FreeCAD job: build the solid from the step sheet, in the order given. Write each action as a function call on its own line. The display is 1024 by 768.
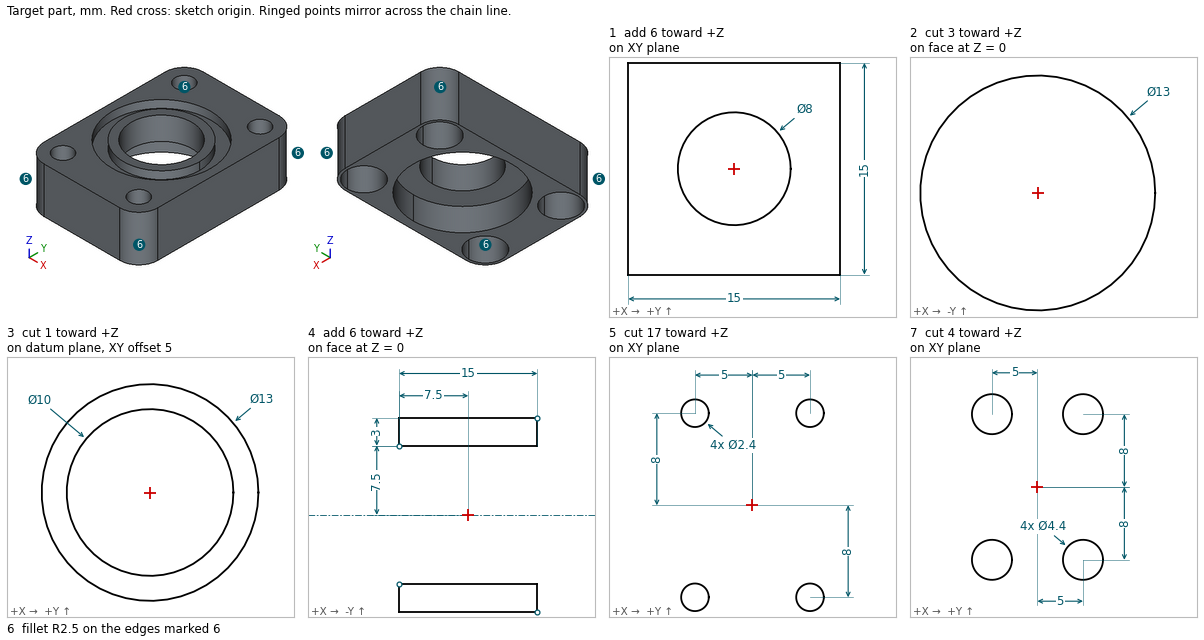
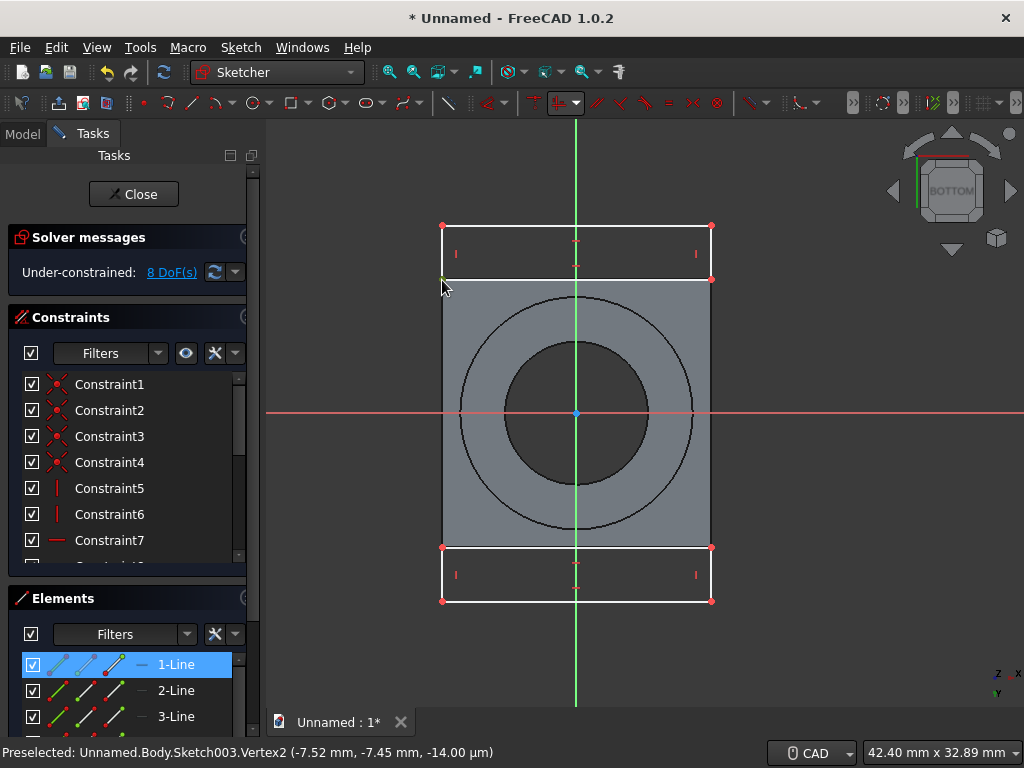
click(442, 548)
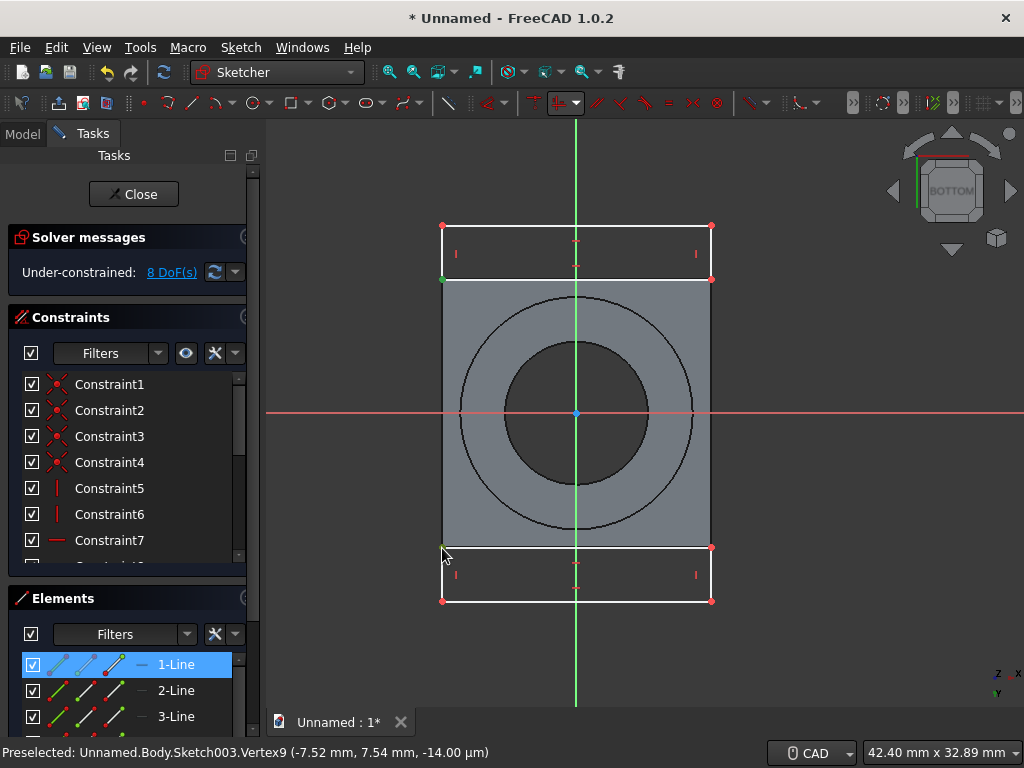
click(334, 413)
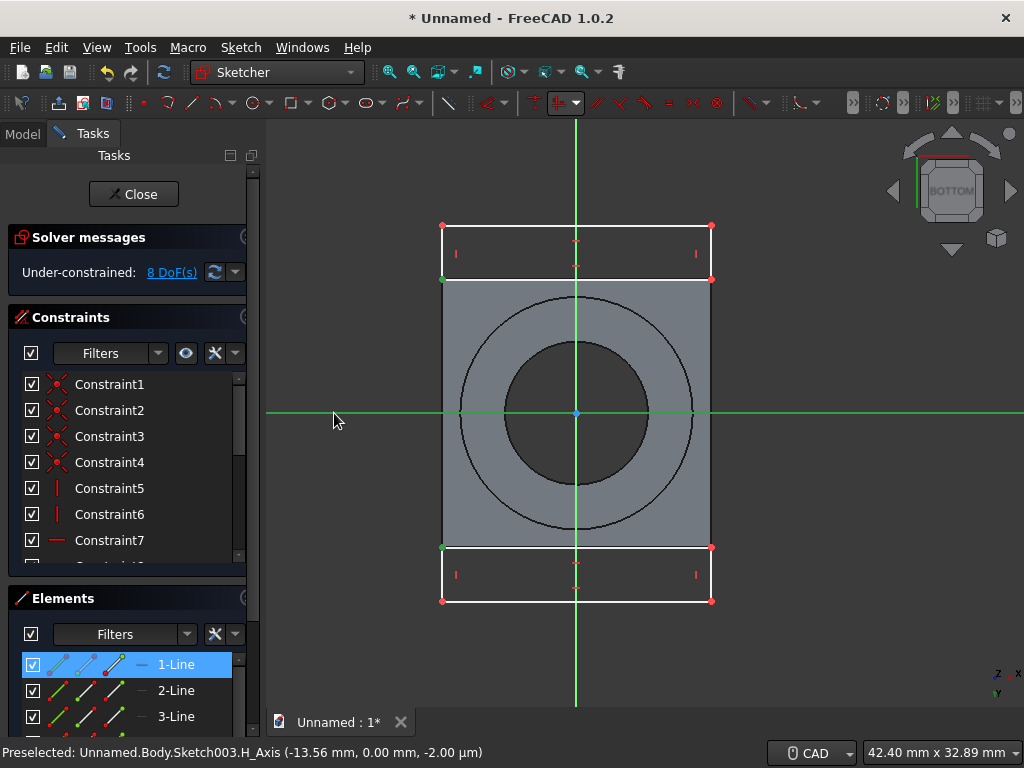
click(694, 104)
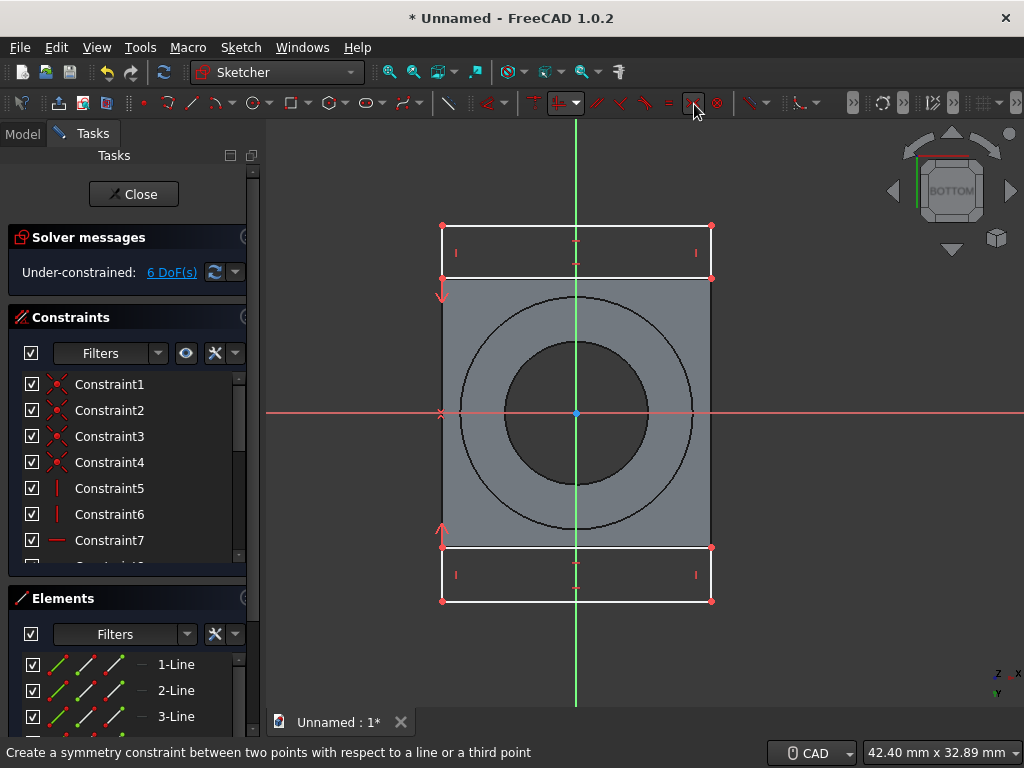
click(711, 226)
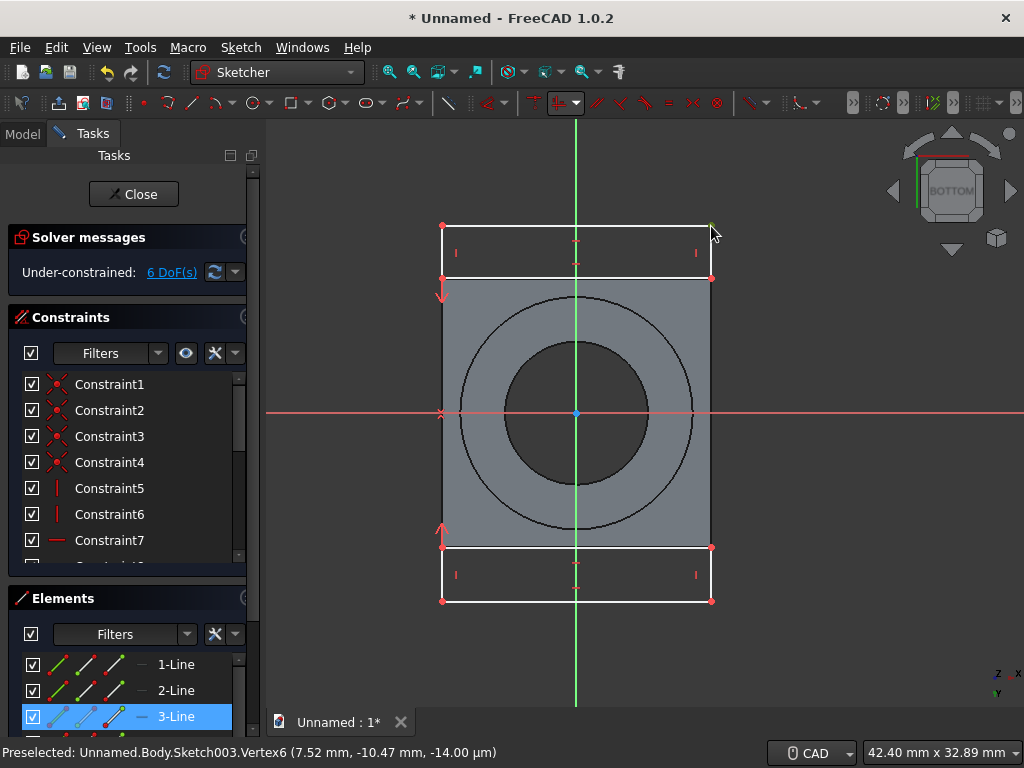
click(711, 602)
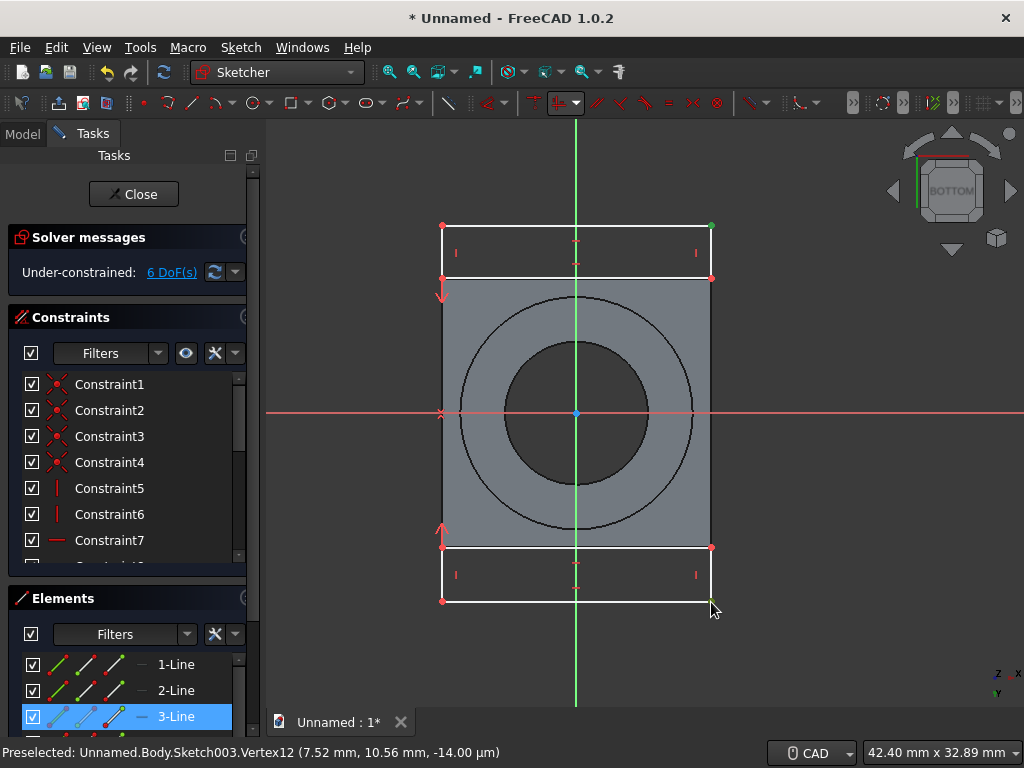
click(334, 413)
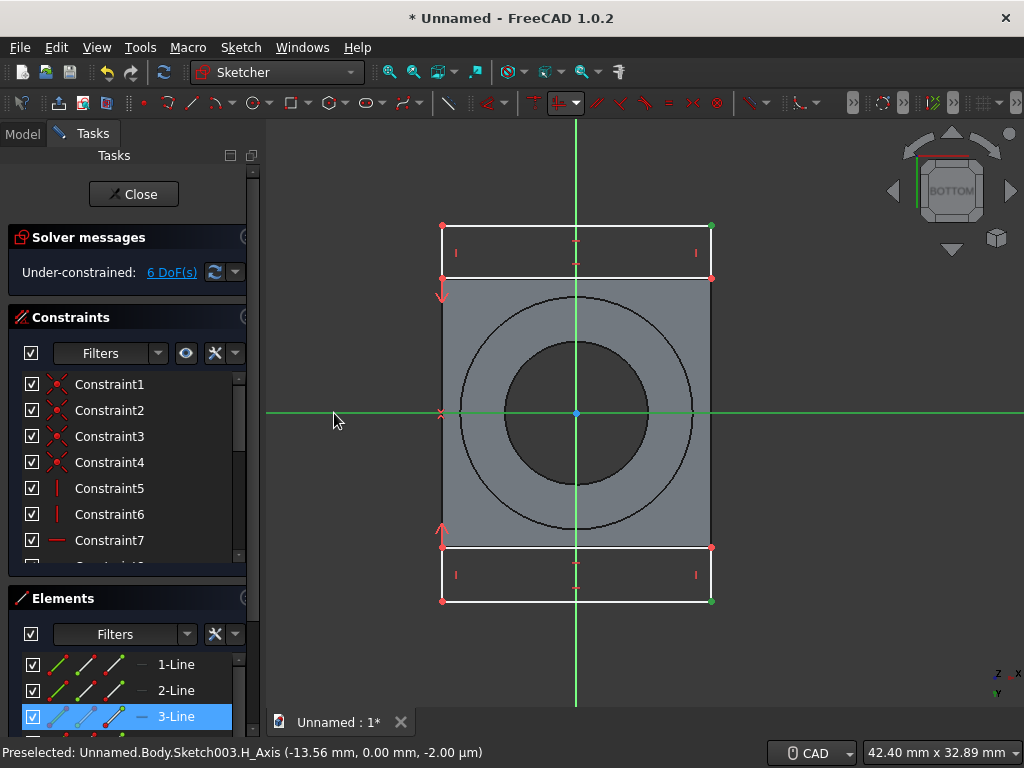
key(s)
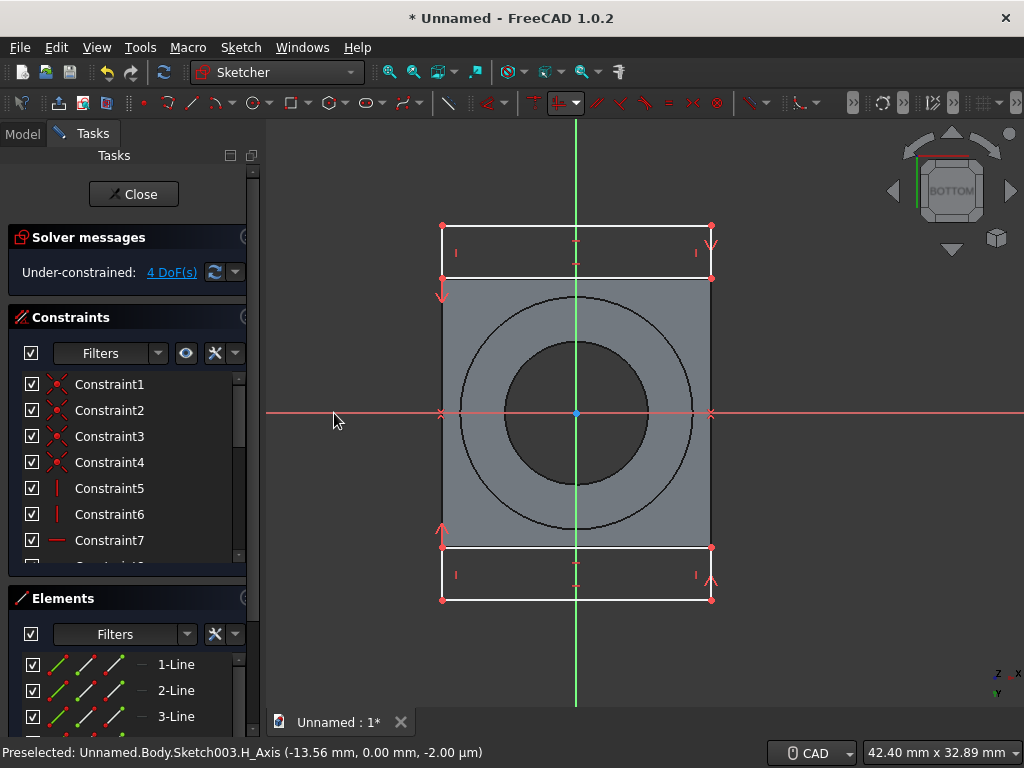
click(488, 104)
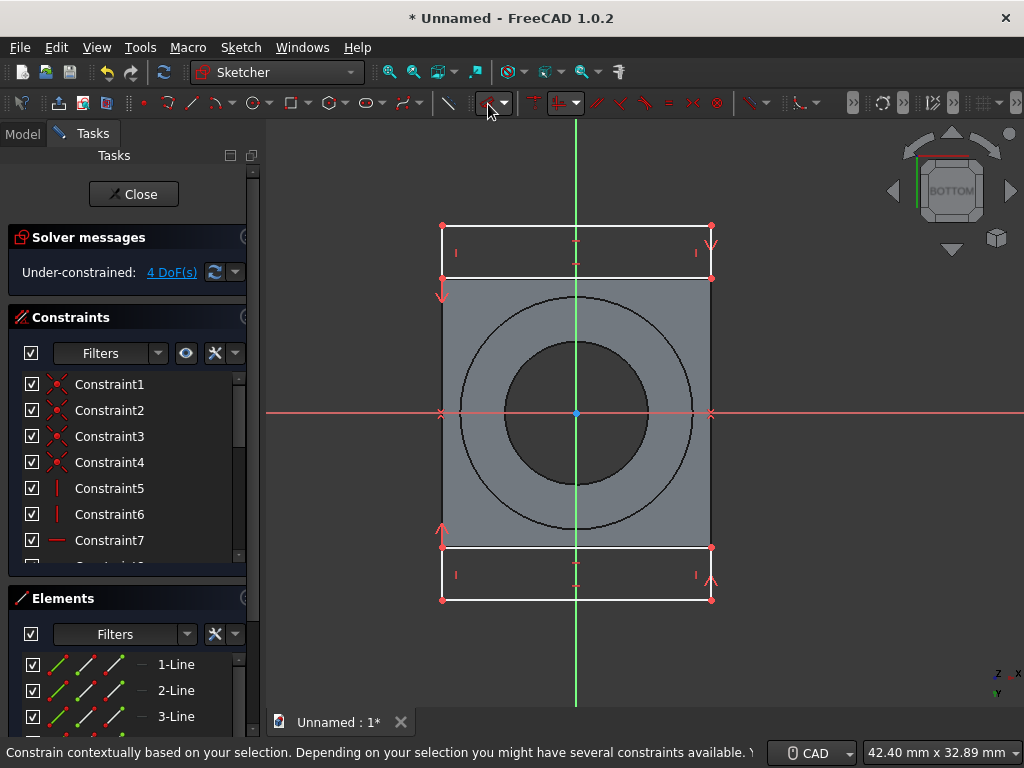
click(442, 242)
click(408, 252)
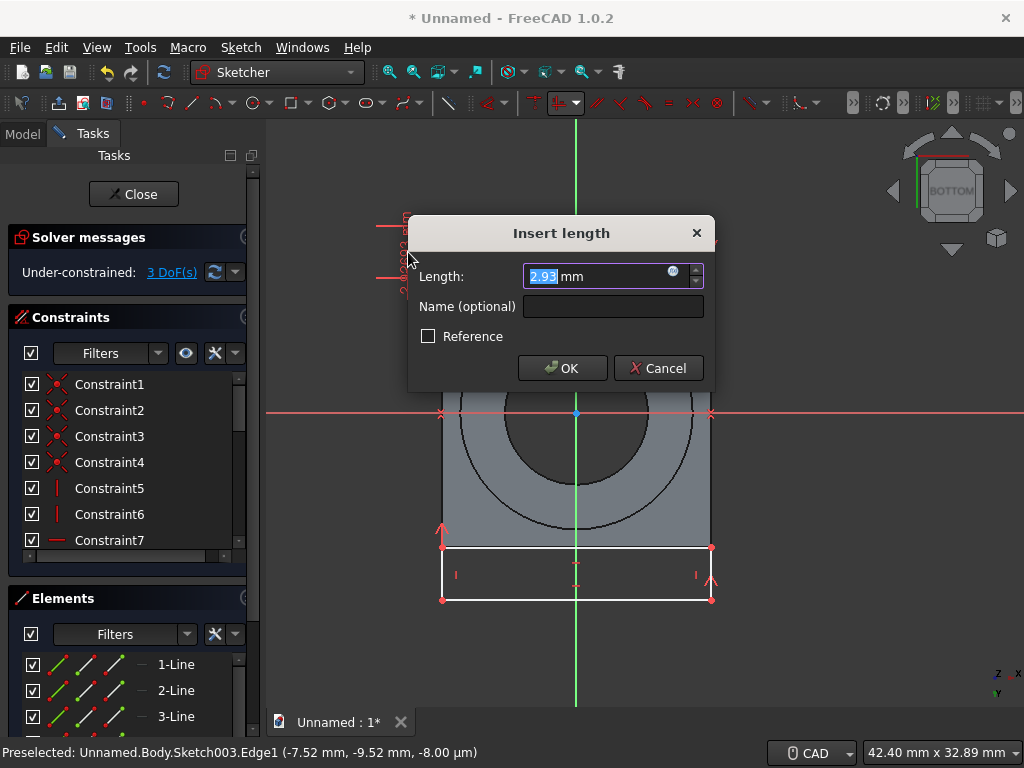
text(3)
key(Return)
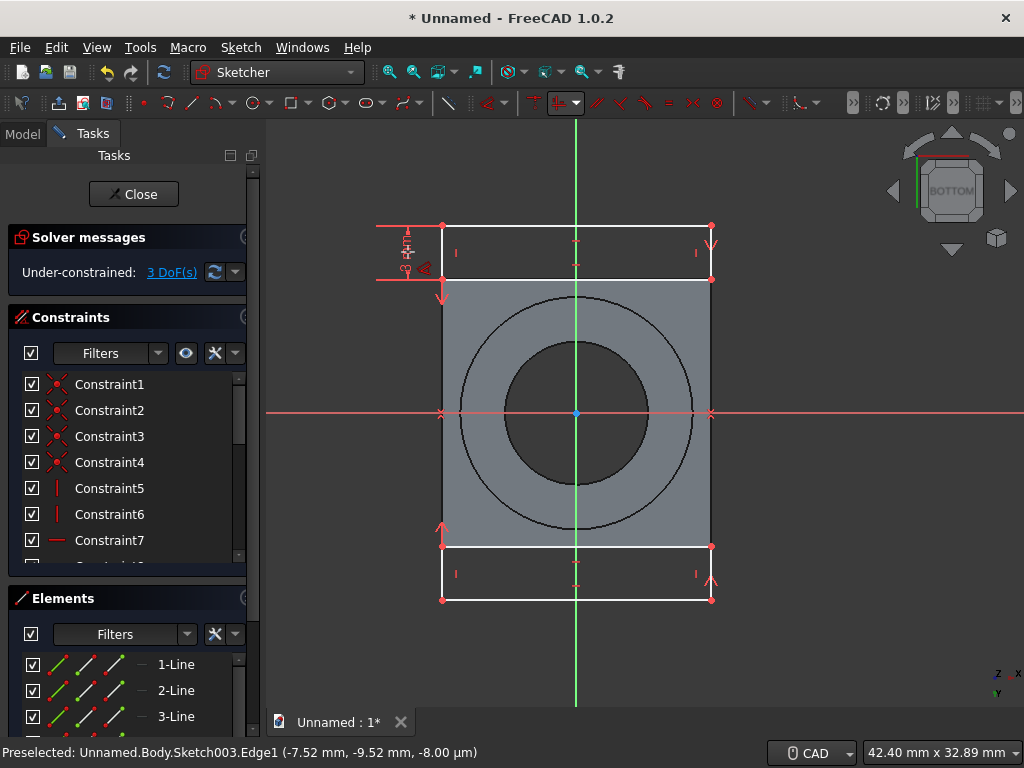
click(523, 280)
click(515, 246)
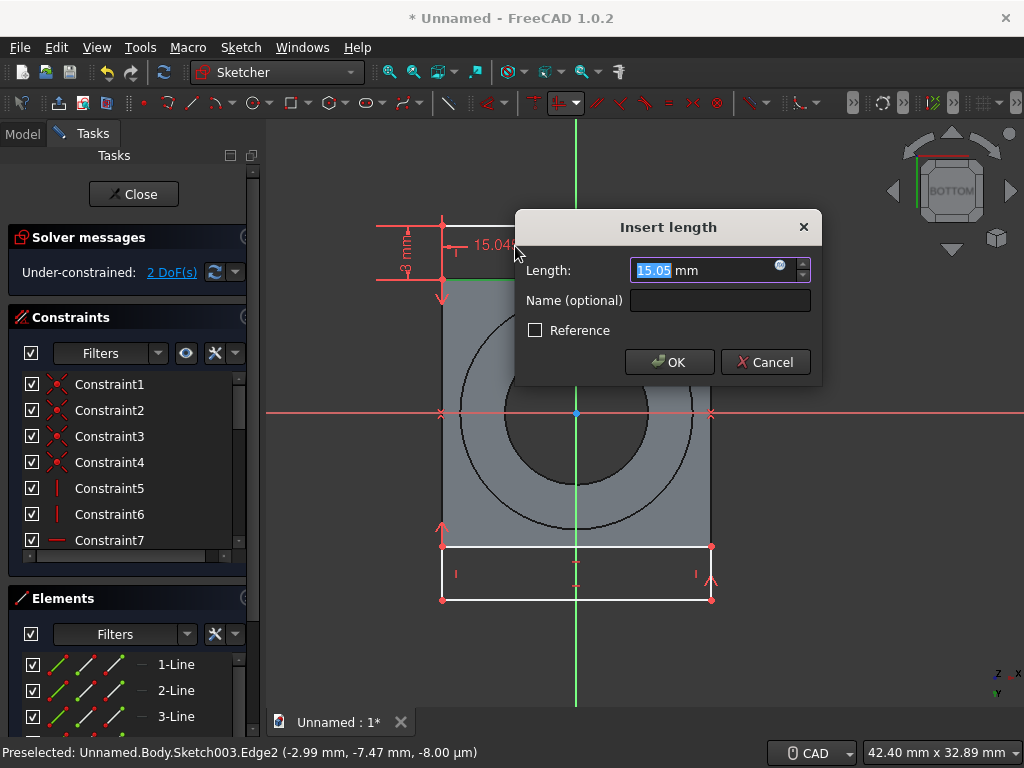
text(15)
key(Return)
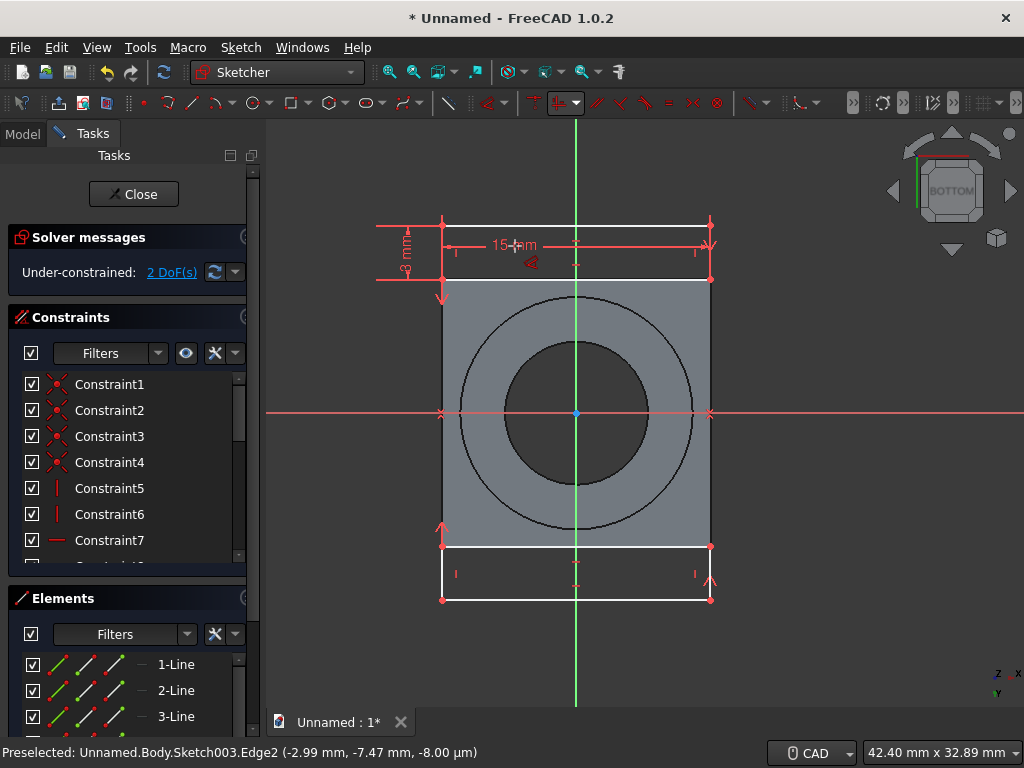
click(442, 226)
click(509, 192)